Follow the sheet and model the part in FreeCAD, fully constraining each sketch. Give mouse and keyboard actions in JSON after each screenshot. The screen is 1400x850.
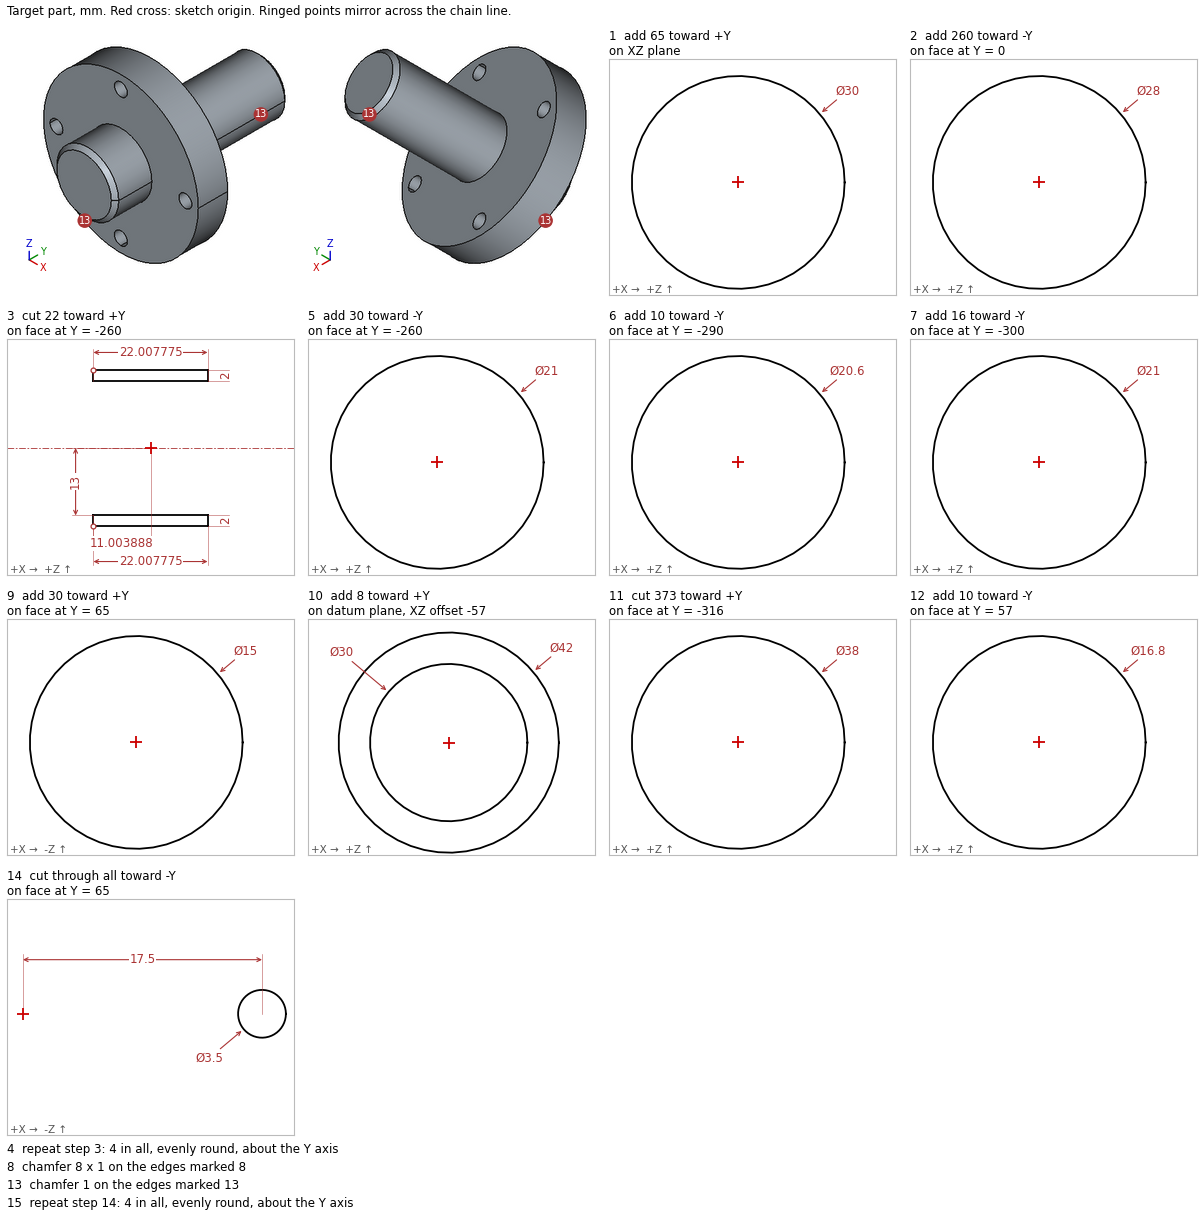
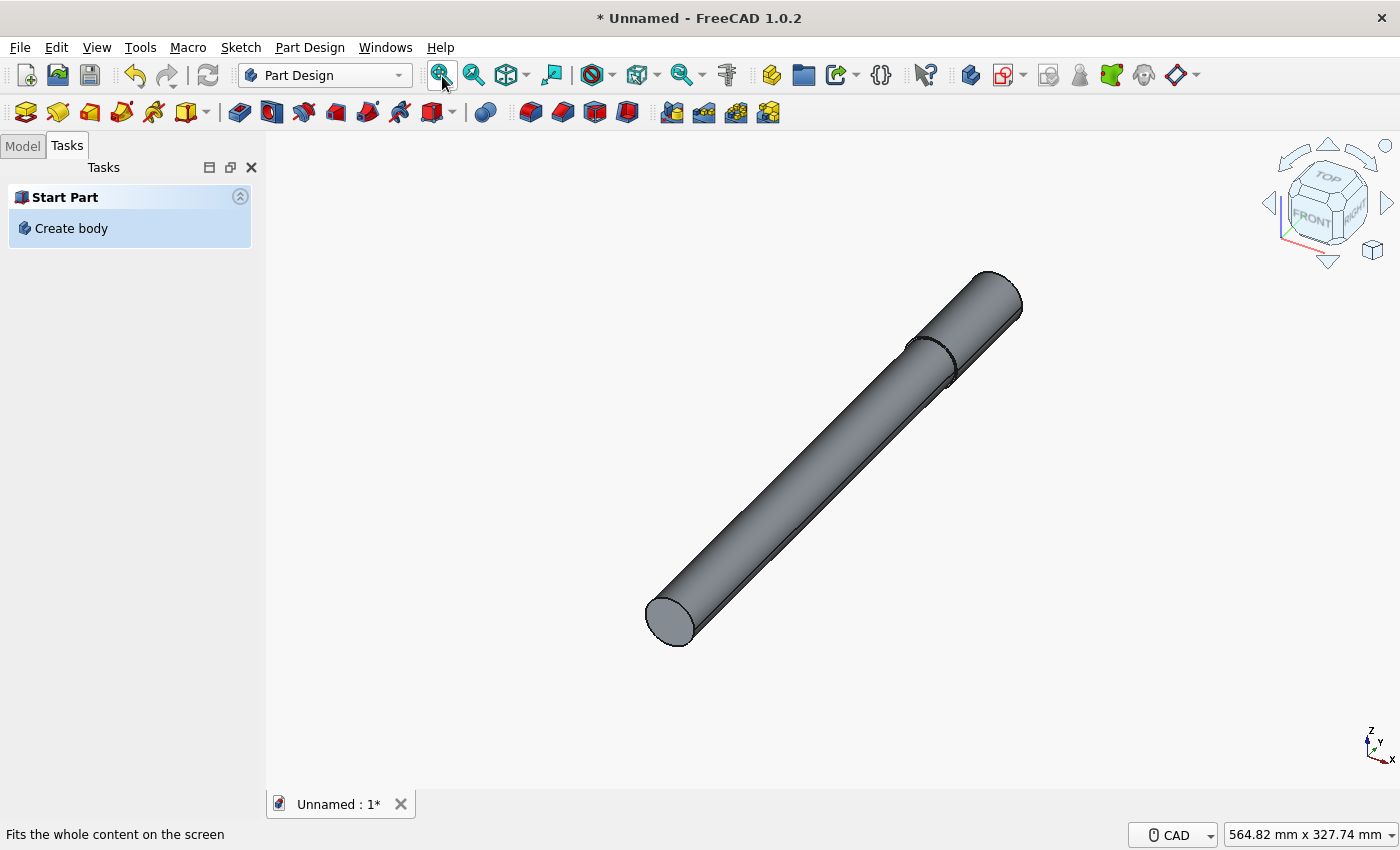
{"action": "left_click", "coordinate": [670, 621]}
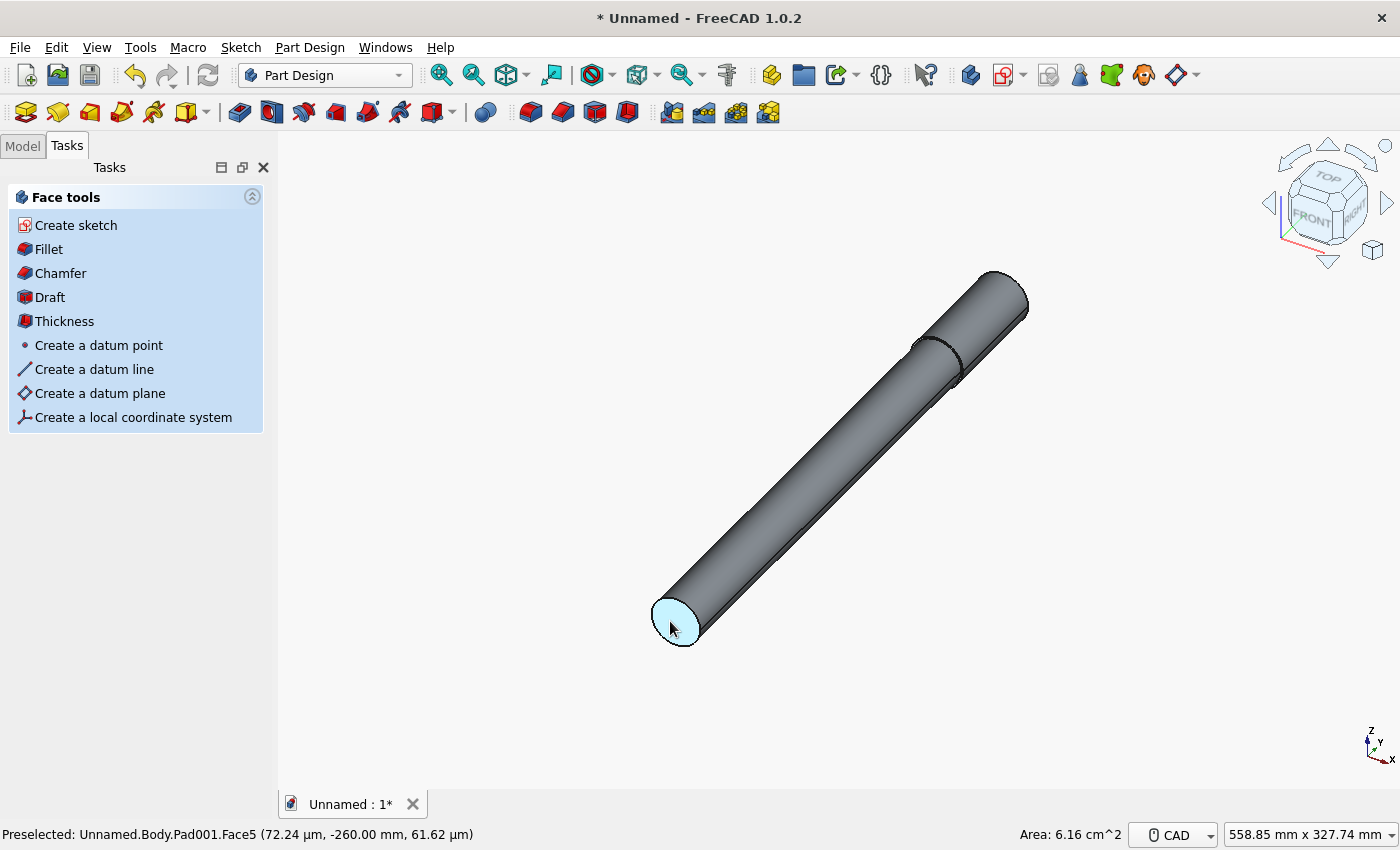
{"action": "left_click", "coordinate": [1004, 76]}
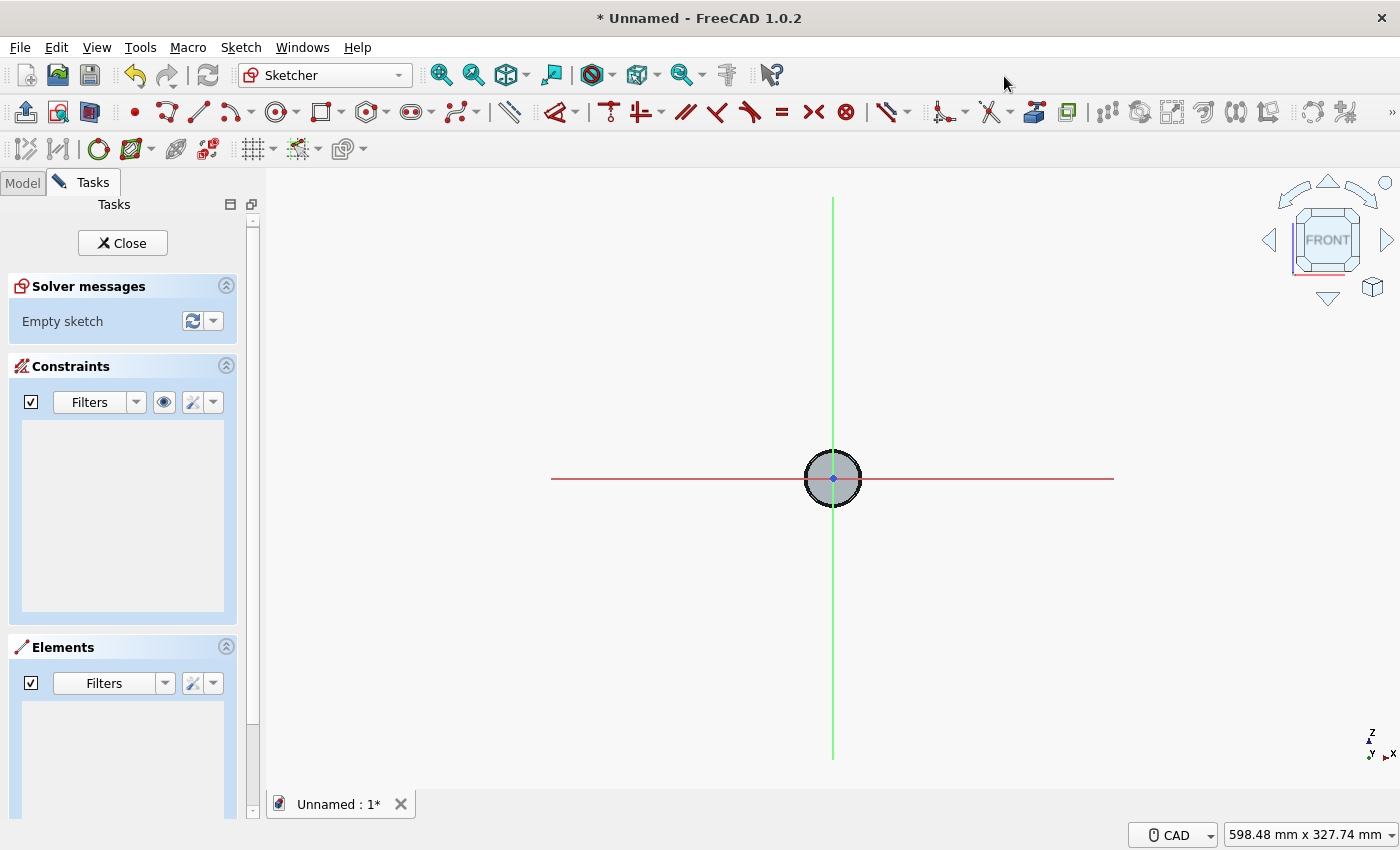
{"action": "scroll", "coordinate": [844, 478], "scroll_direction": "up", "scroll_amount": 10}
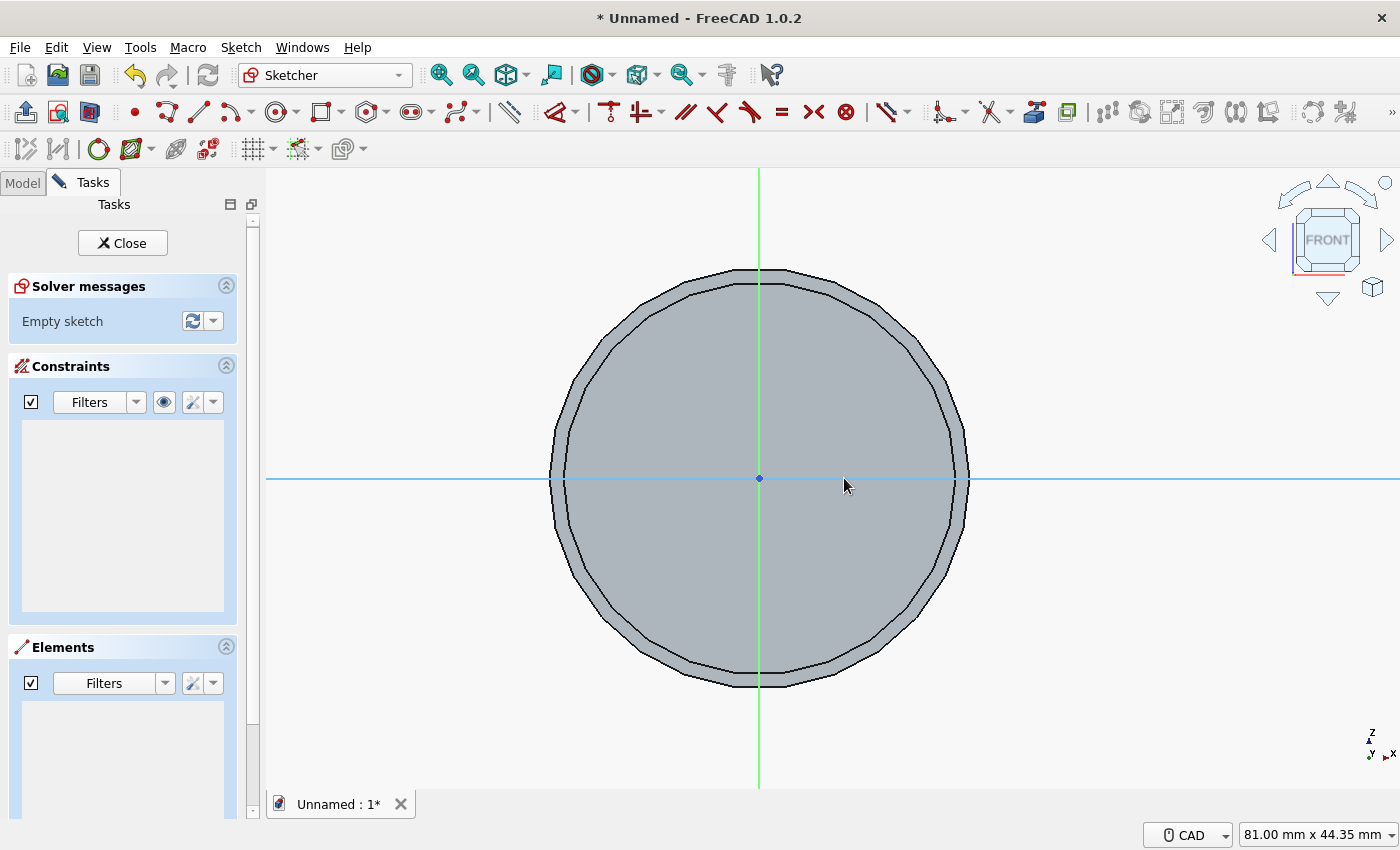
{"action": "left_click", "coordinate": [322, 112]}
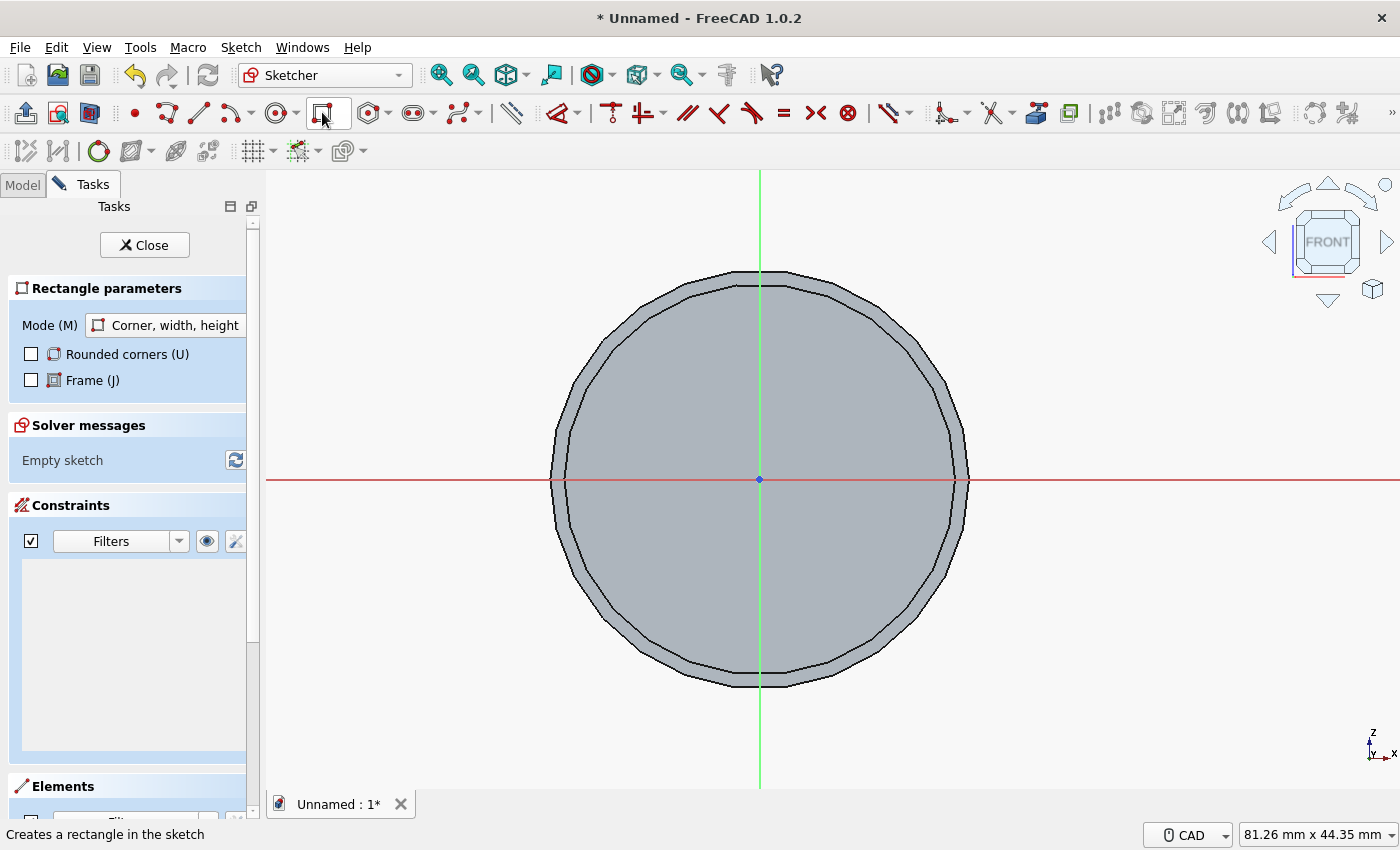
{"action": "left_click", "coordinate": [606, 661]}
{"action": "mouse_move", "coordinate": [913, 689]}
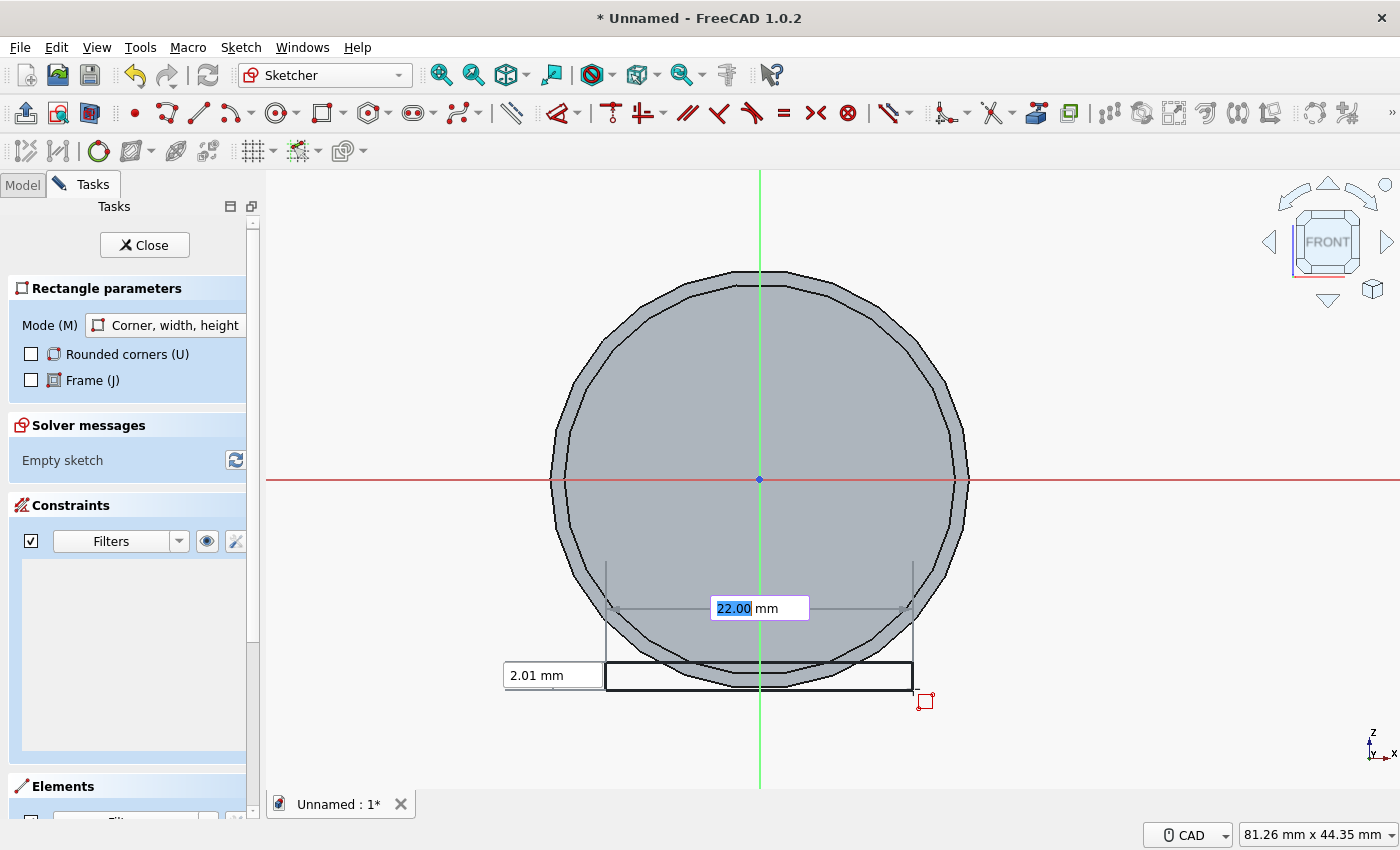
{"action": "type", "text": "22.007775"}
{"action": "key", "text": "Tab"}
{"action": "type", "text": "2"}
{"action": "key", "text": "Return"}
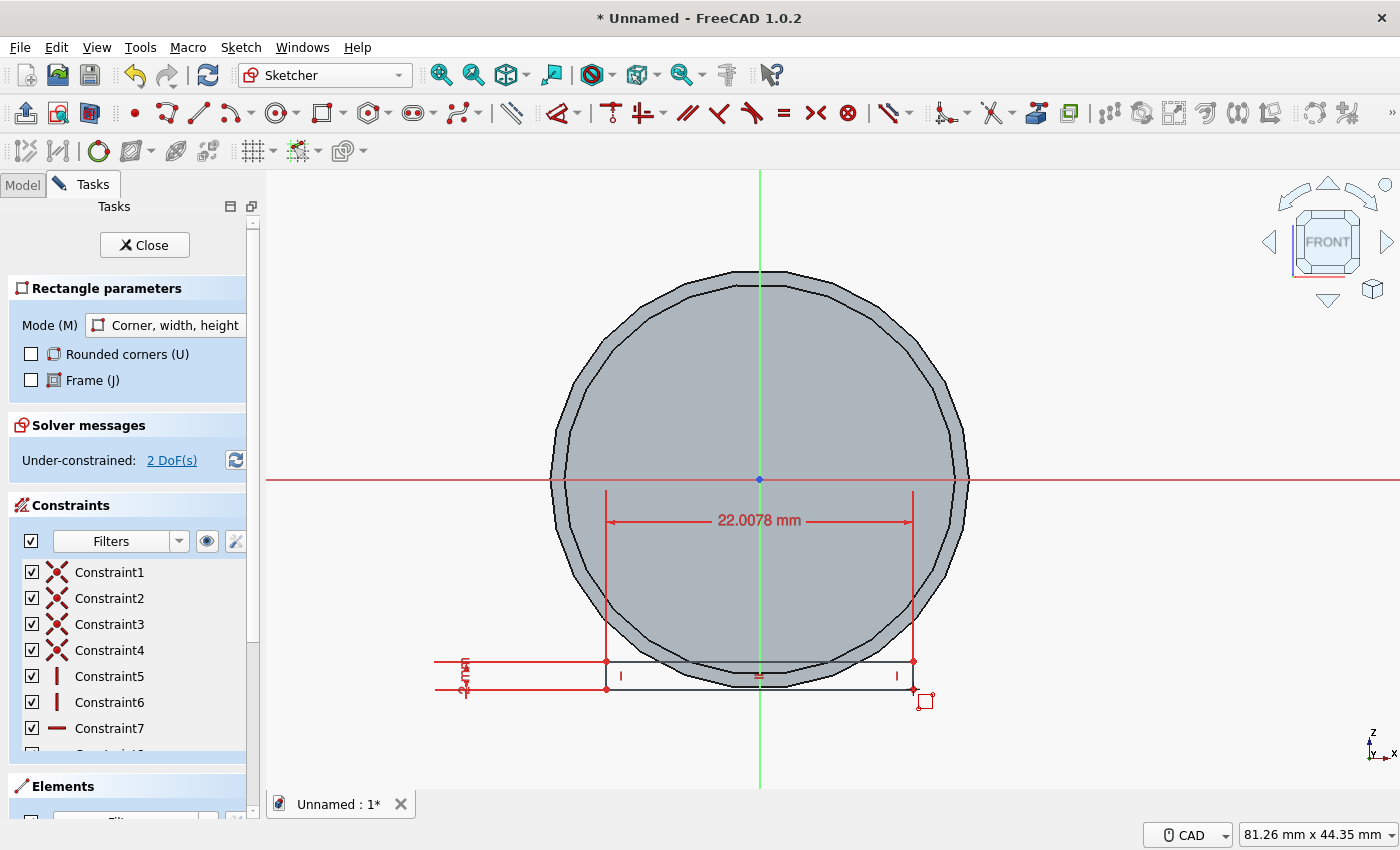
{"action": "left_click", "coordinate": [606, 270]}
{"action": "mouse_move", "coordinate": [913, 298]}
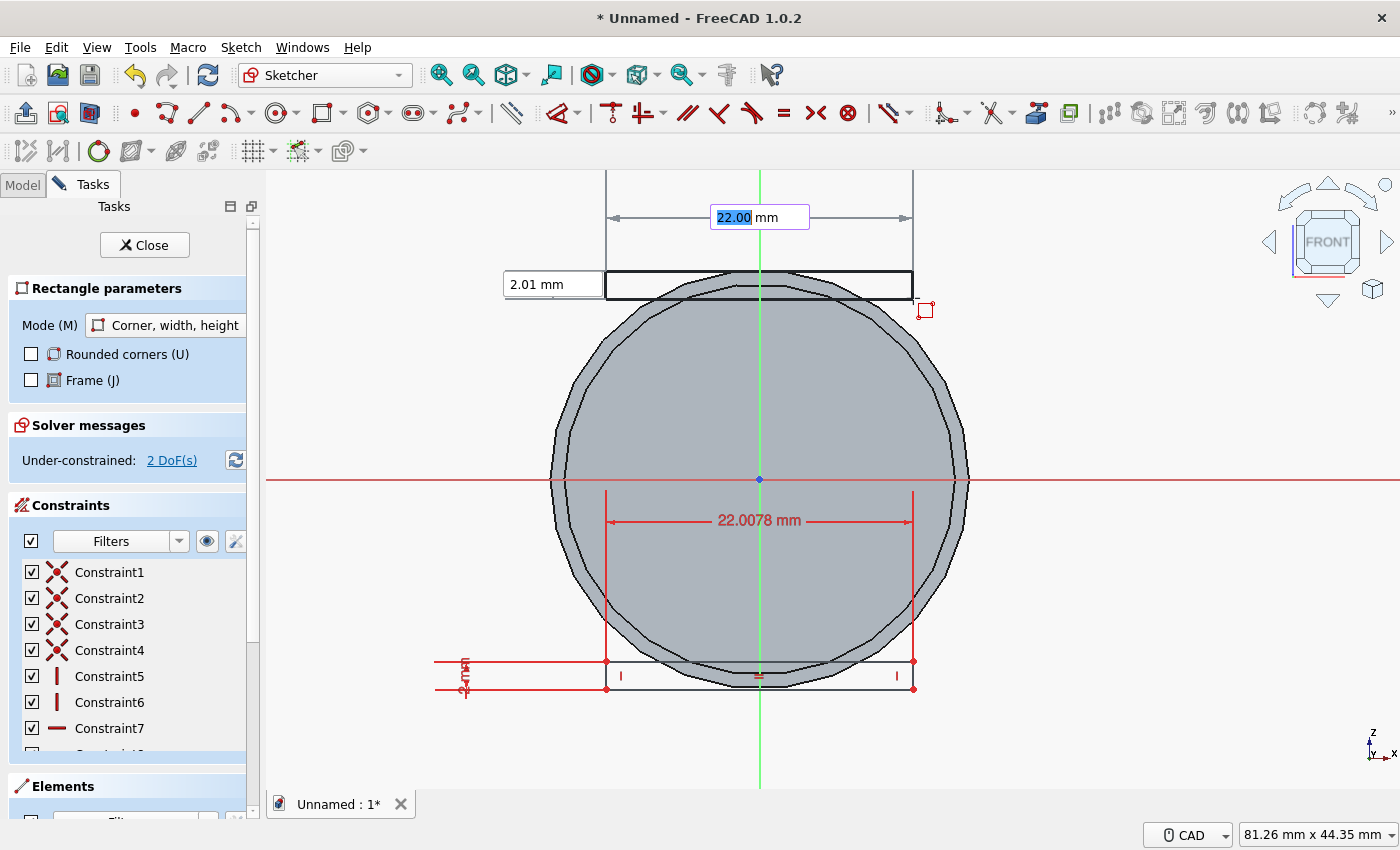
{"action": "type", "text": "22.007775"}
{"action": "key", "text": "Tab"}
{"action": "type", "text": "2"}
{"action": "key", "text": "Return"}
{"action": "key", "text": "Escape"}